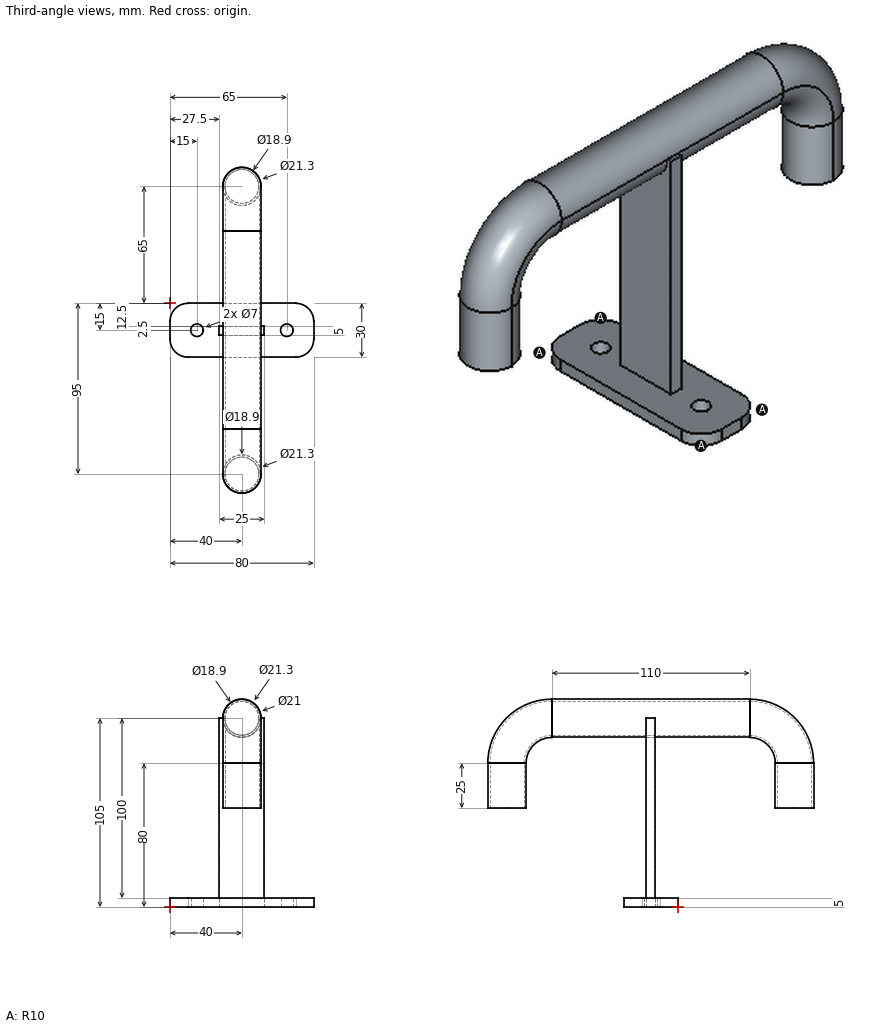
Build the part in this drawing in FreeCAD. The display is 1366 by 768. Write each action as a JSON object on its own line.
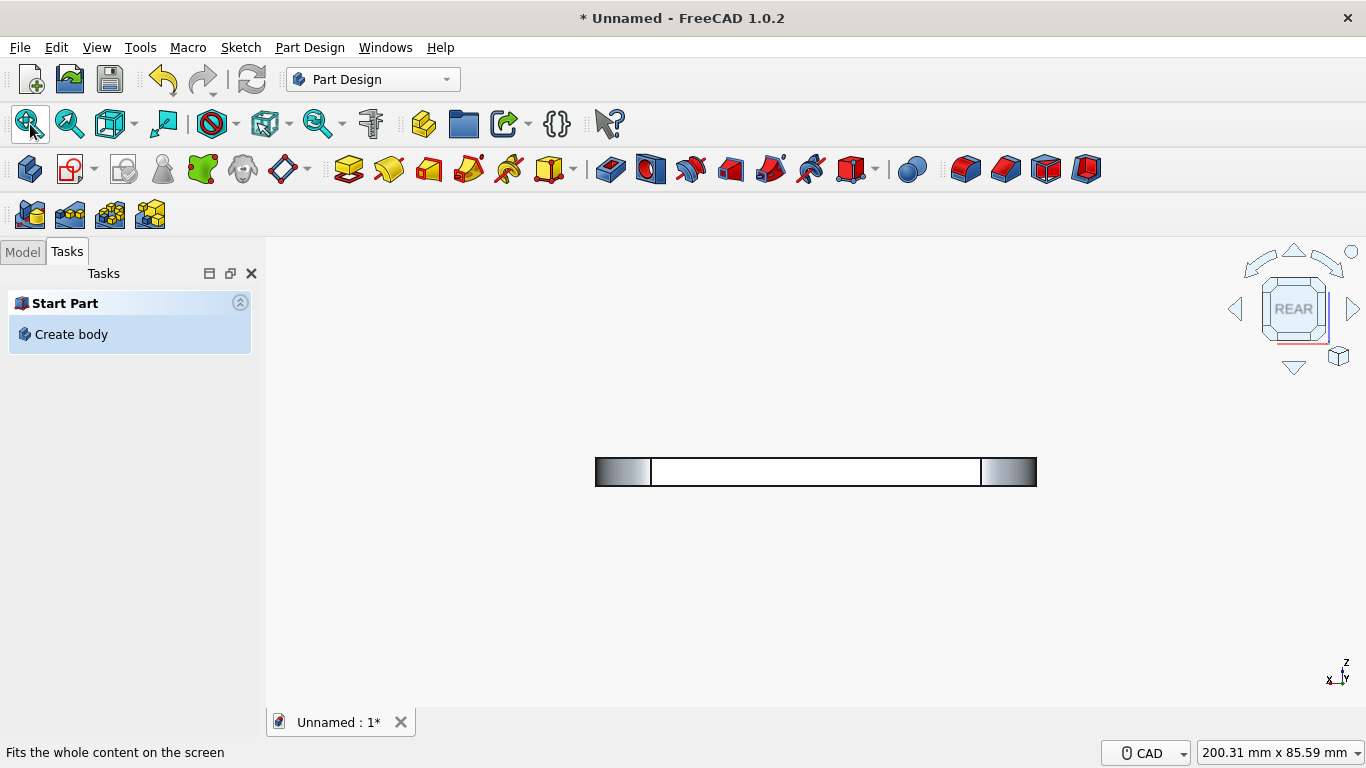
{"action": "left_click", "coordinate": [30, 170]}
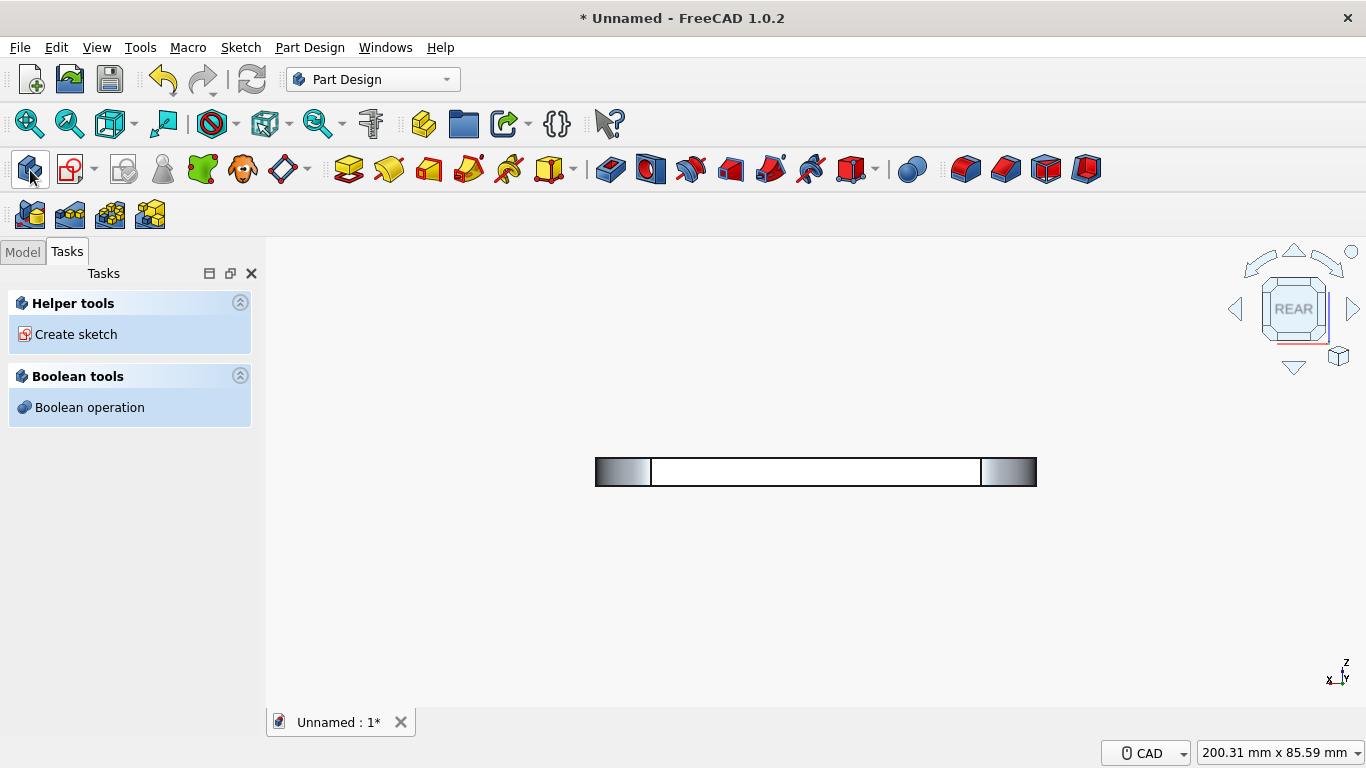
{"action": "left_click", "coordinate": [23, 251]}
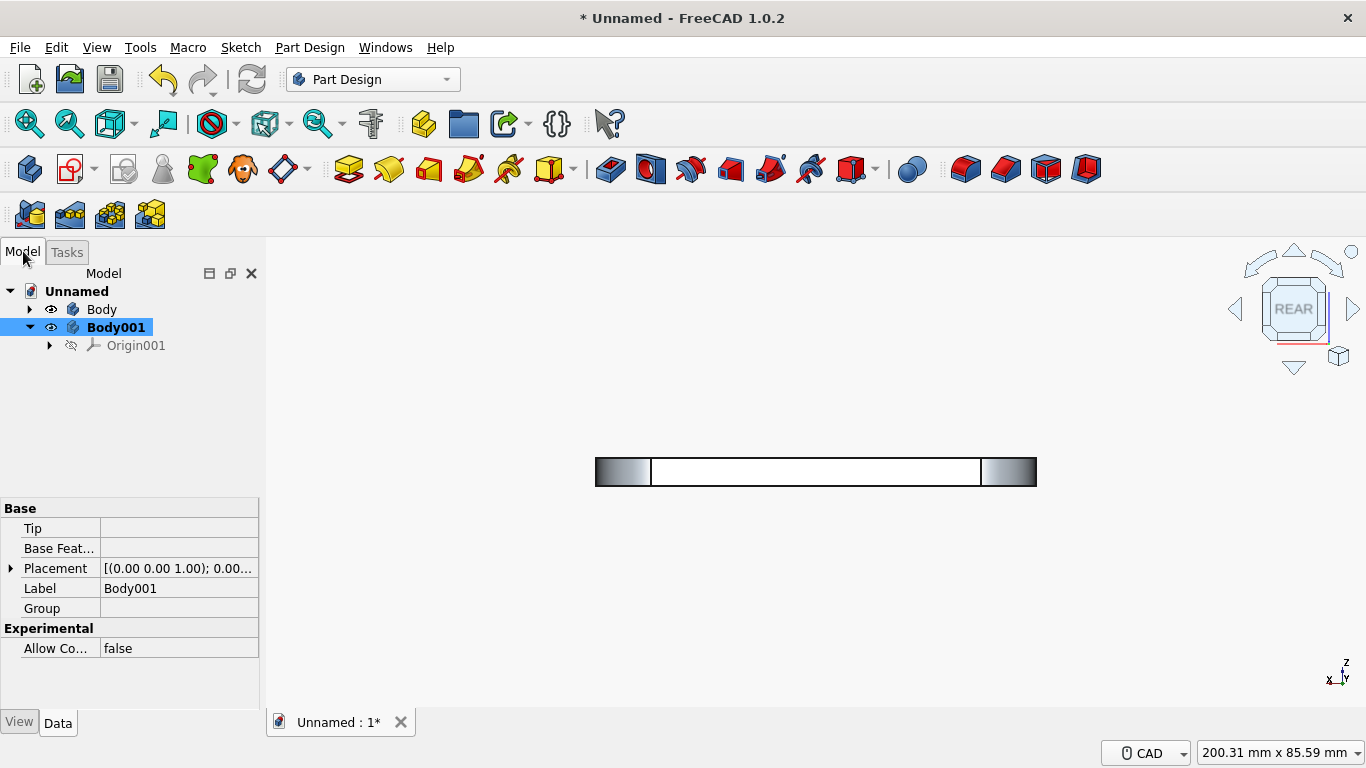
{"action": "left_click", "coordinate": [50, 345]}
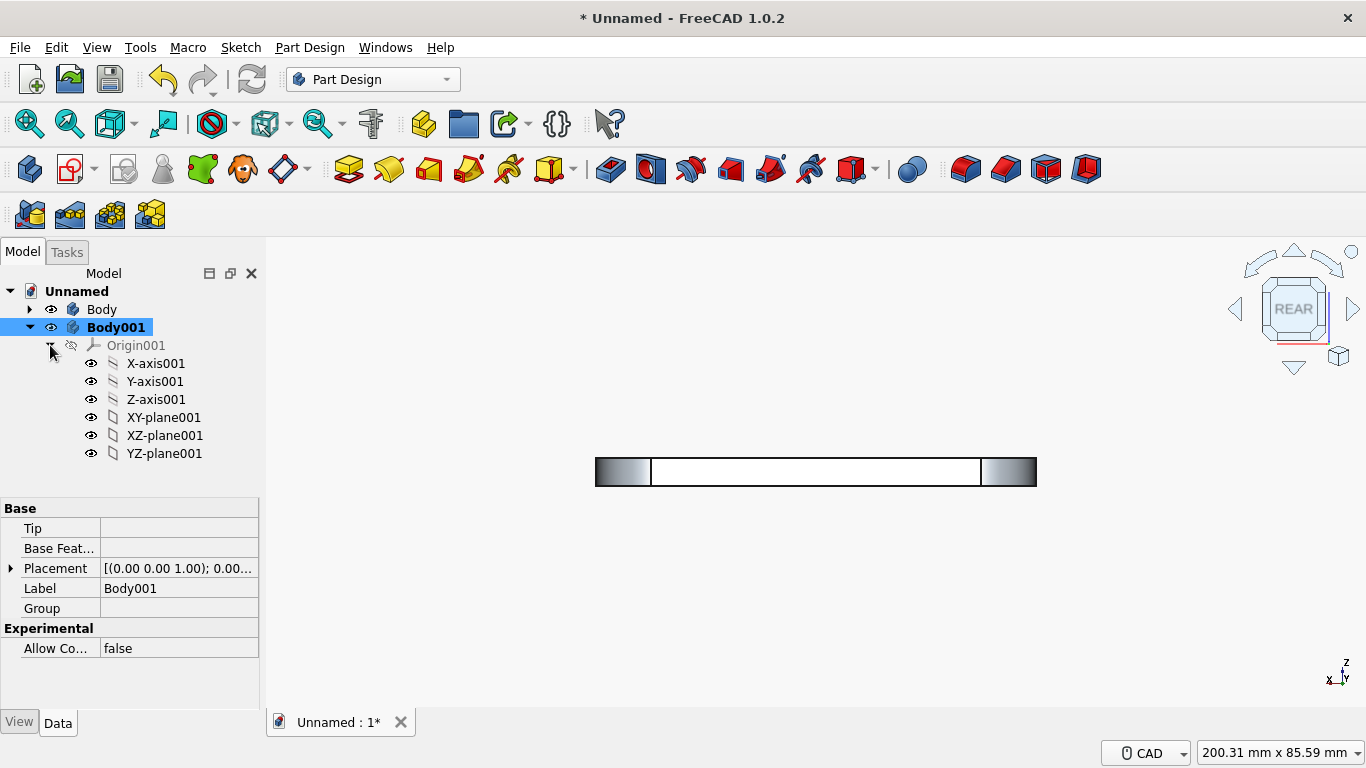
{"action": "left_click", "coordinate": [136, 417]}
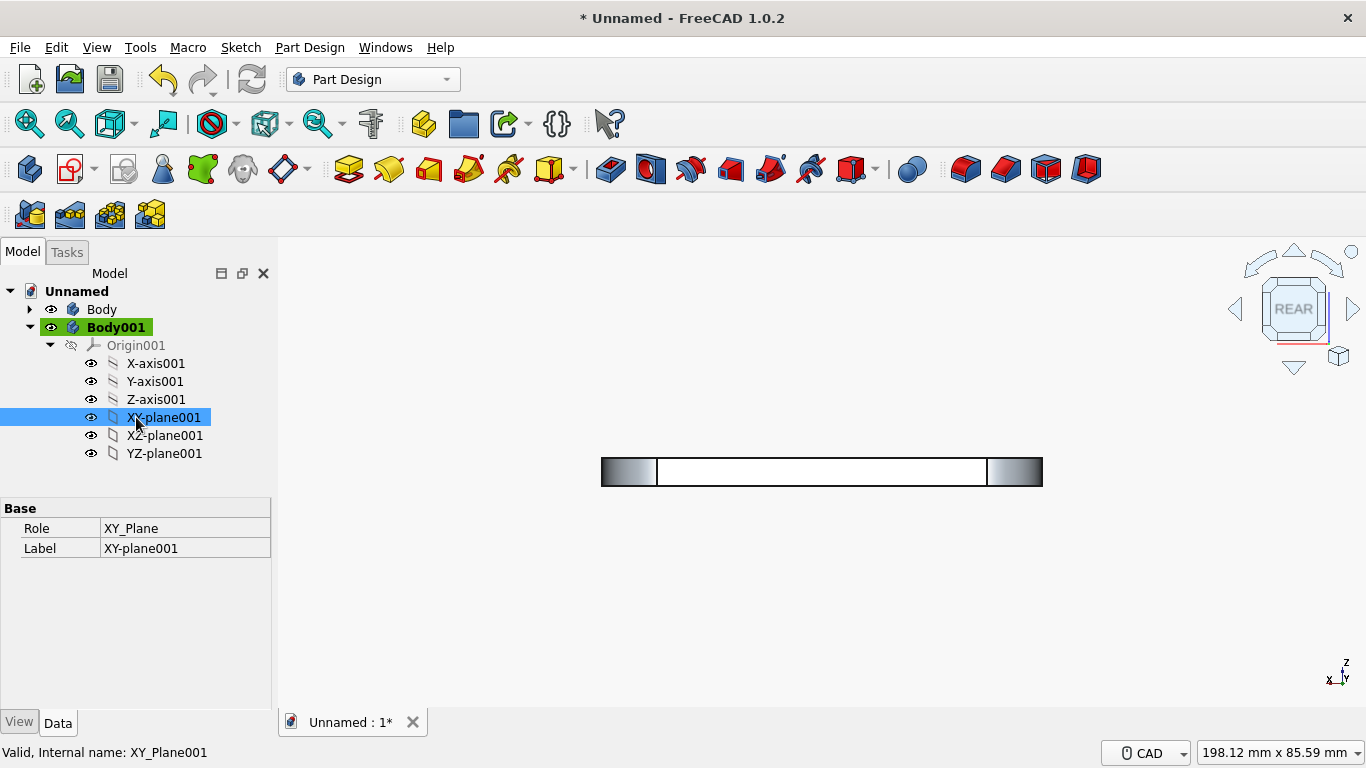
{"action": "left_click", "coordinate": [284, 170]}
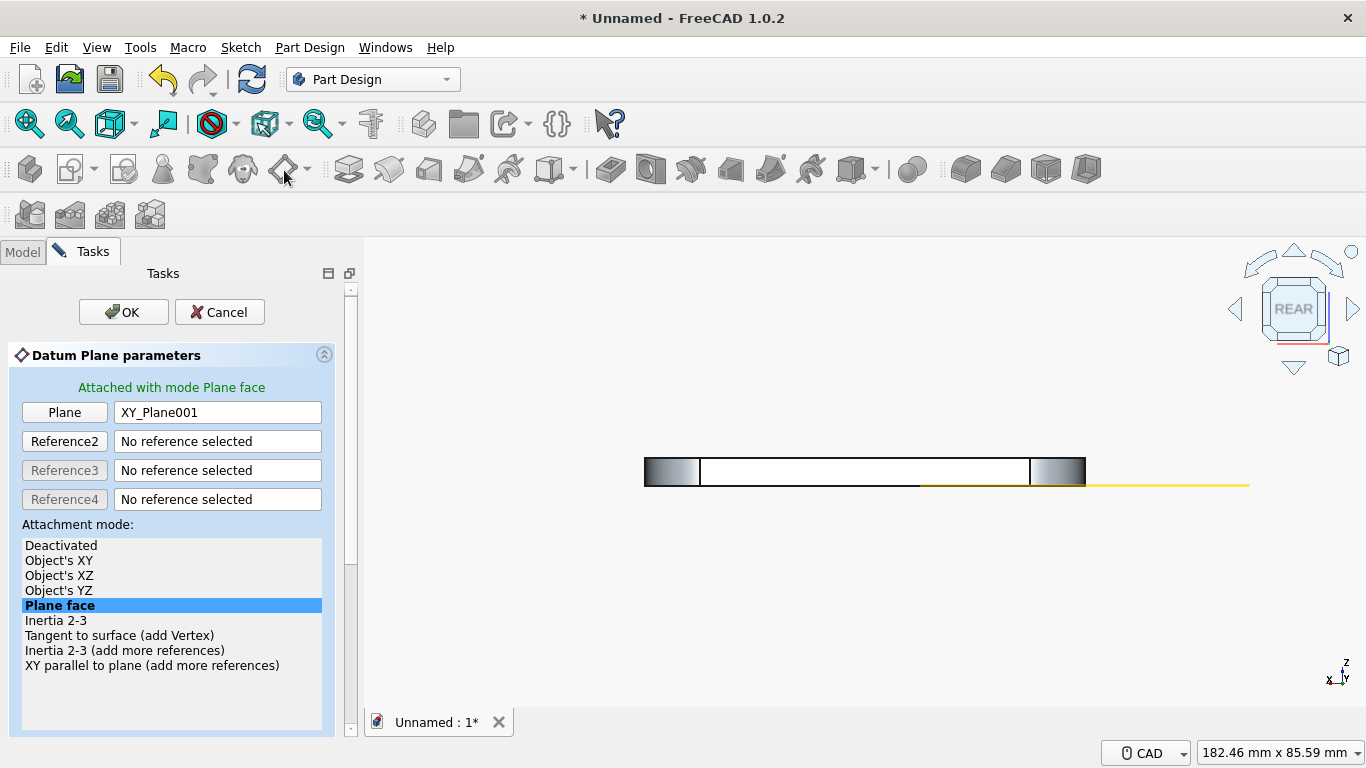
{"action": "scroll", "coordinate": [351, 510], "scroll_direction": "down", "scroll_amount": 3}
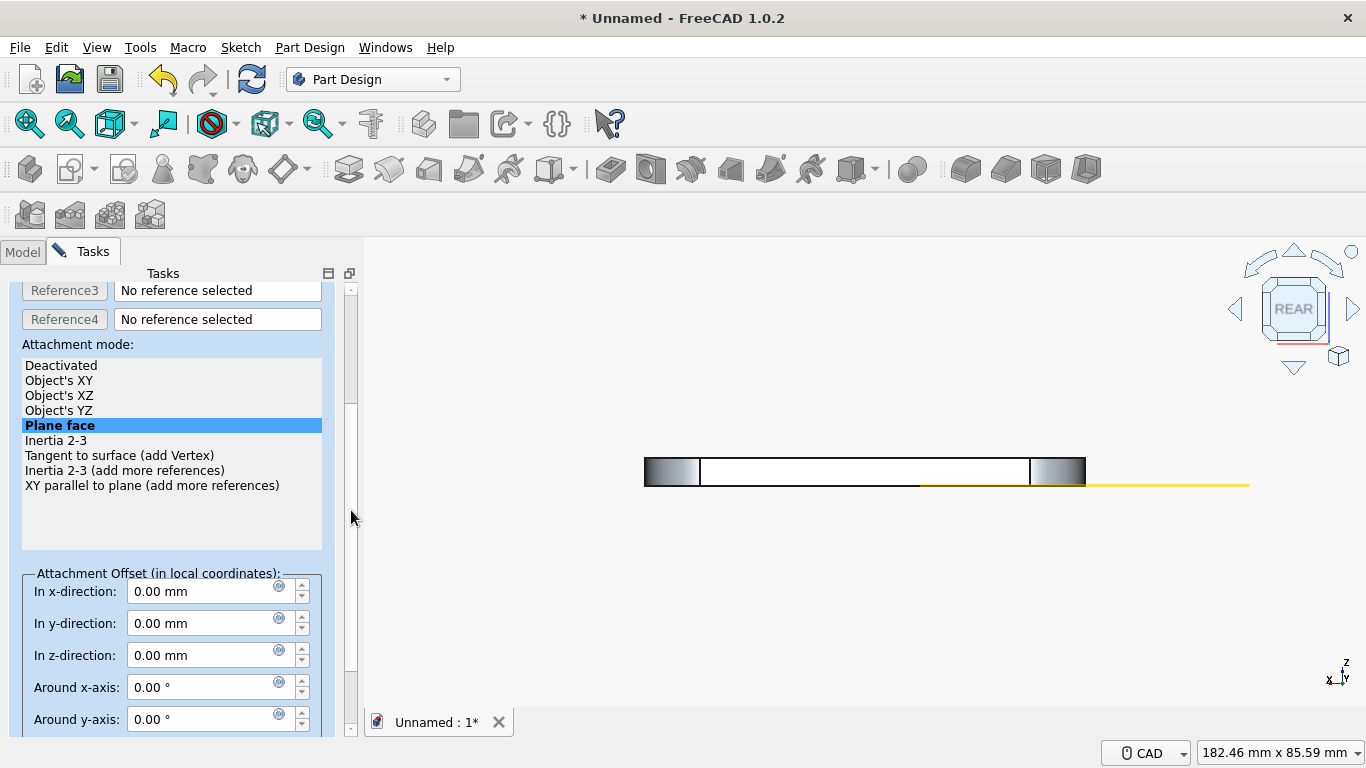
{"action": "triple_click", "coordinate": [210, 655]}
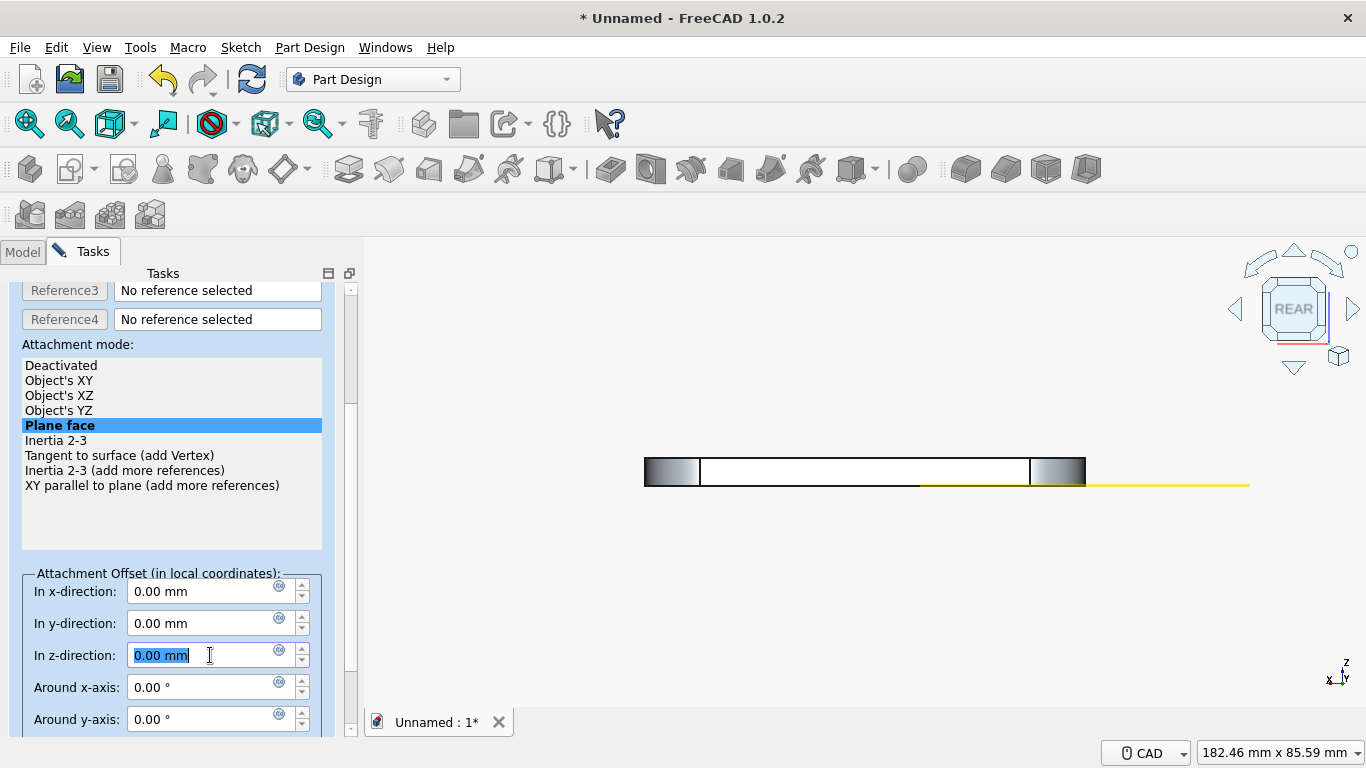
{"action": "type", "text": "5"}
{"action": "key", "text": "Tab"}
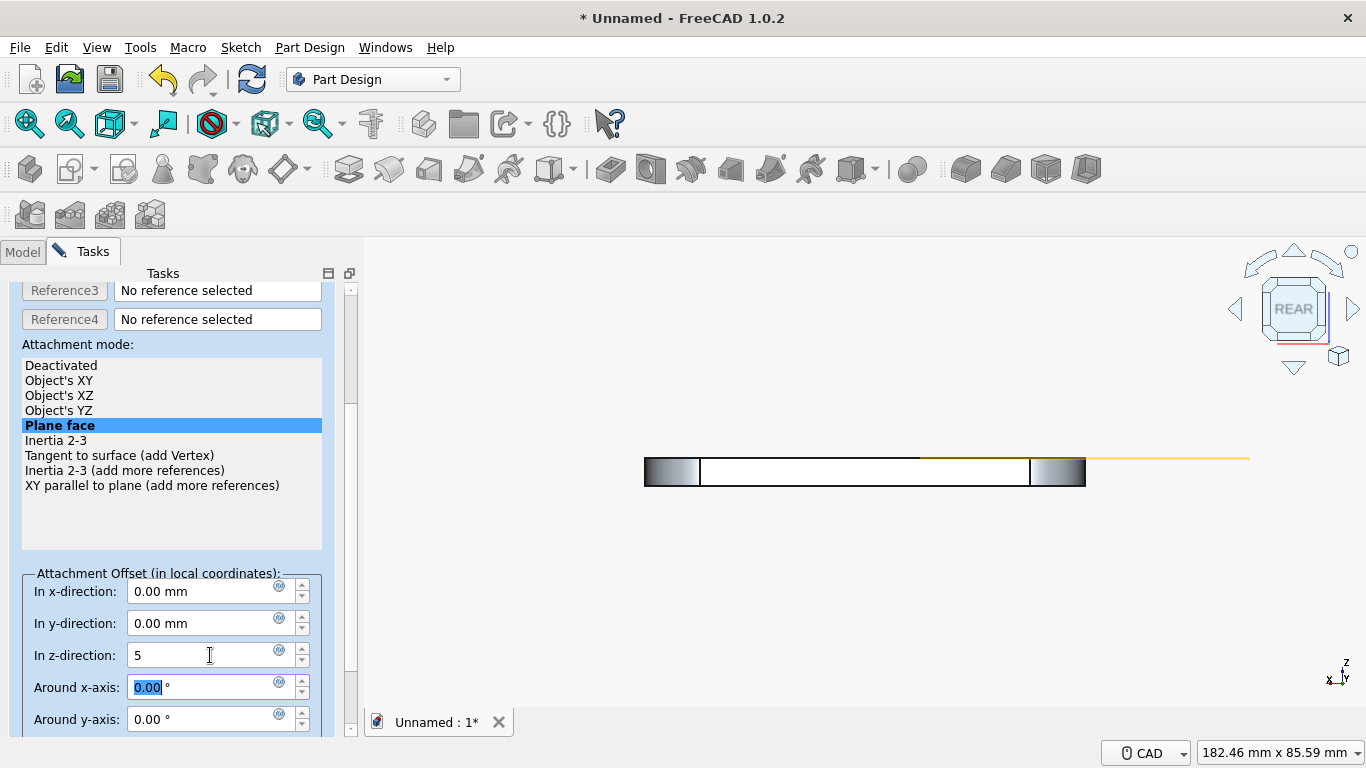
{"action": "scroll", "coordinate": [351, 510], "scroll_direction": "up", "scroll_amount": 4}